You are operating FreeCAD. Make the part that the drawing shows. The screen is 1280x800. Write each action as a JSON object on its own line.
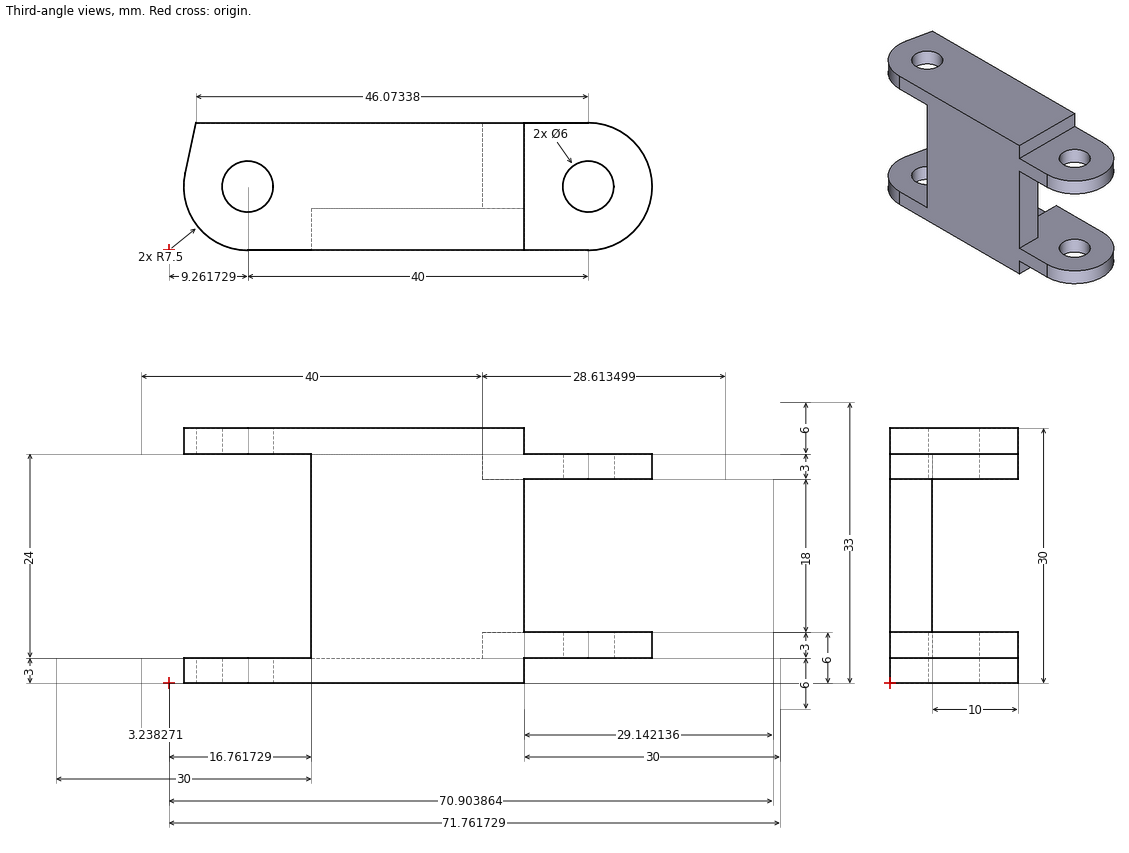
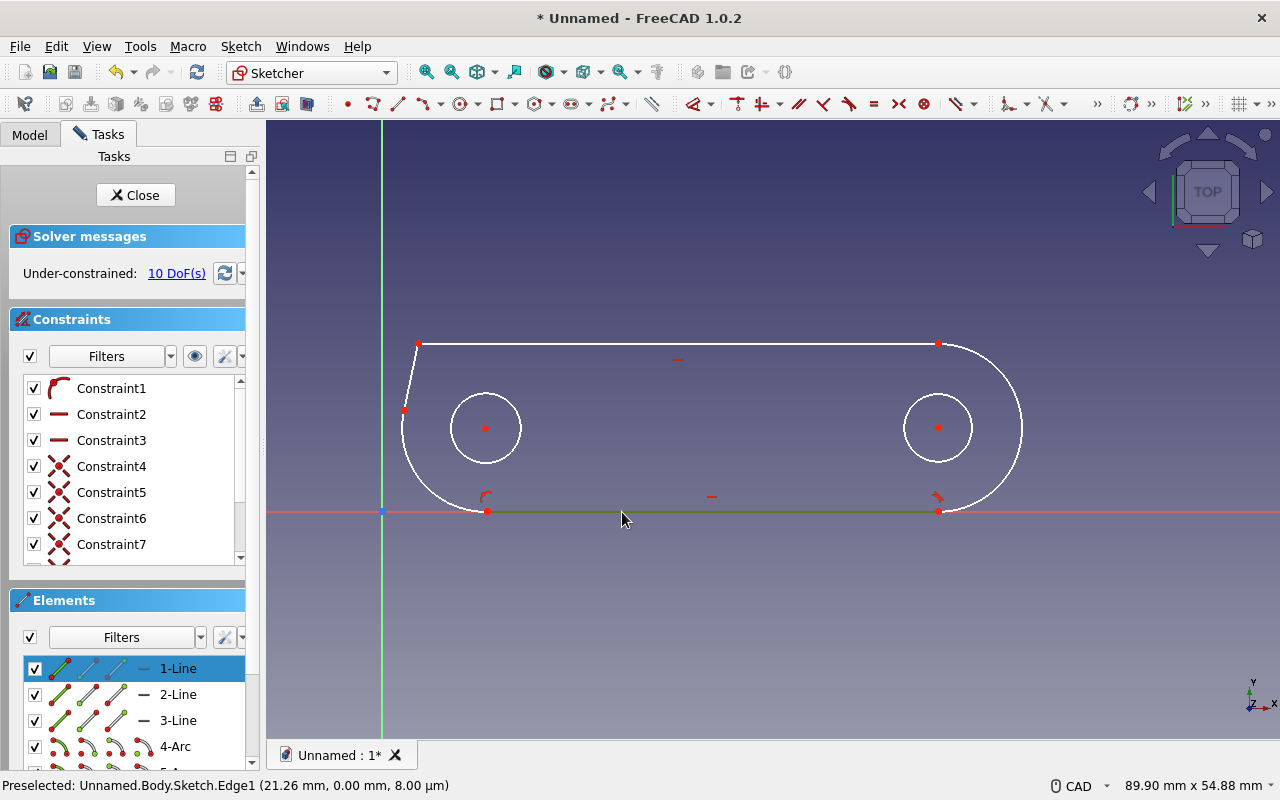
{"action": "left_click", "coordinate": [407, 455]}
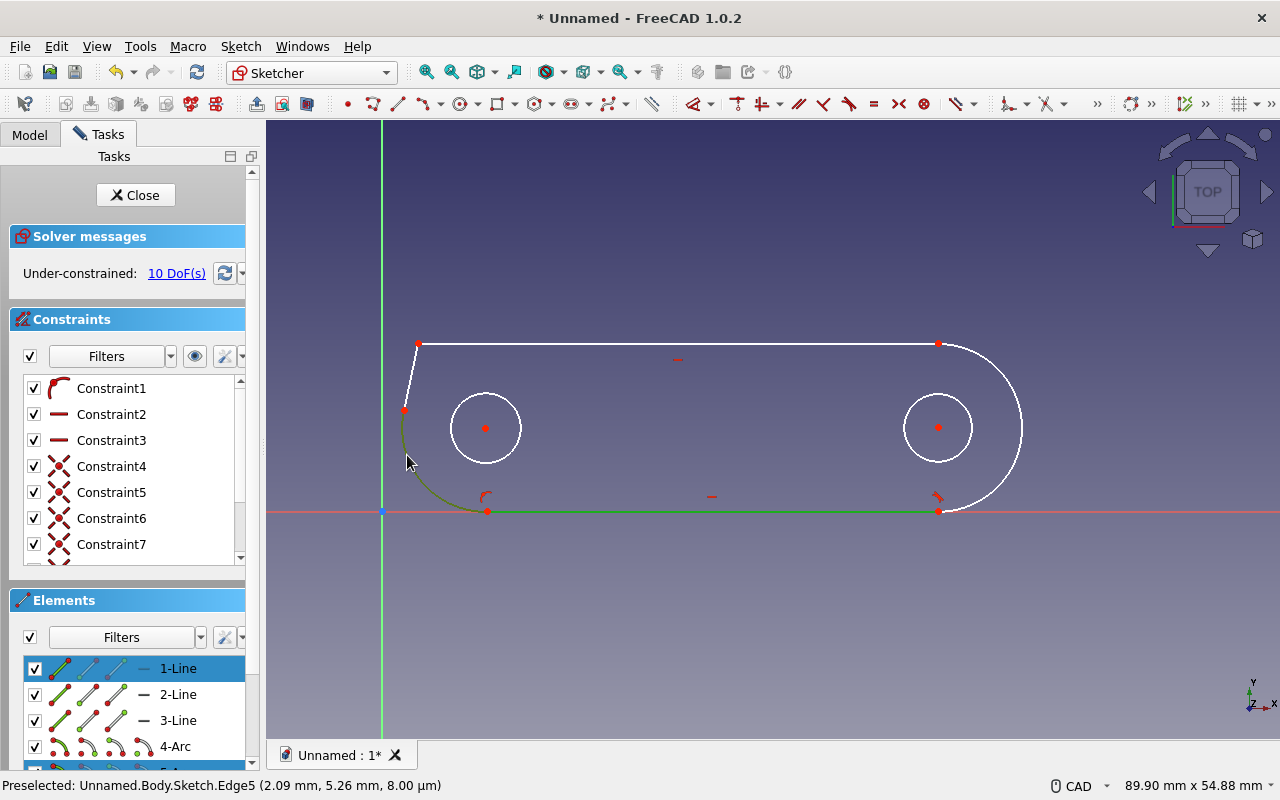
{"action": "left_click", "coordinate": [849, 104]}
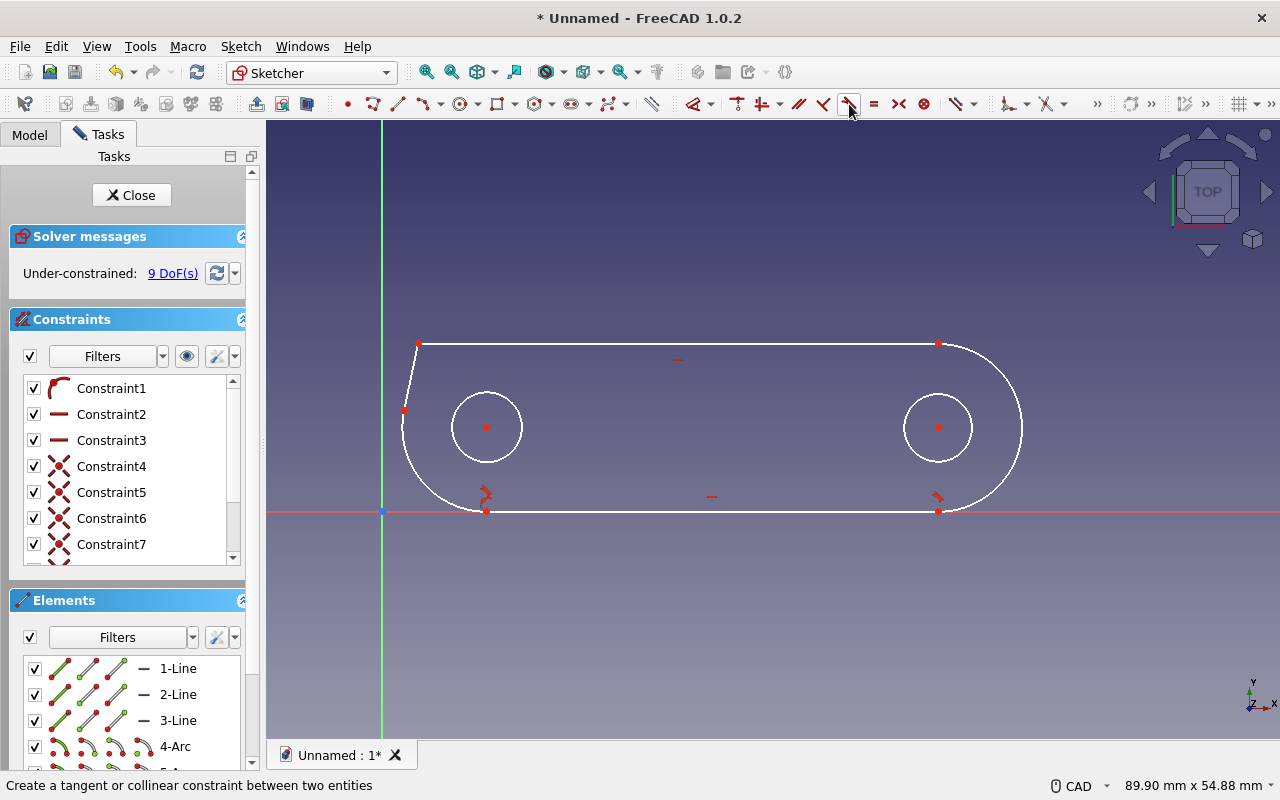
{"action": "left_click", "coordinate": [782, 344]}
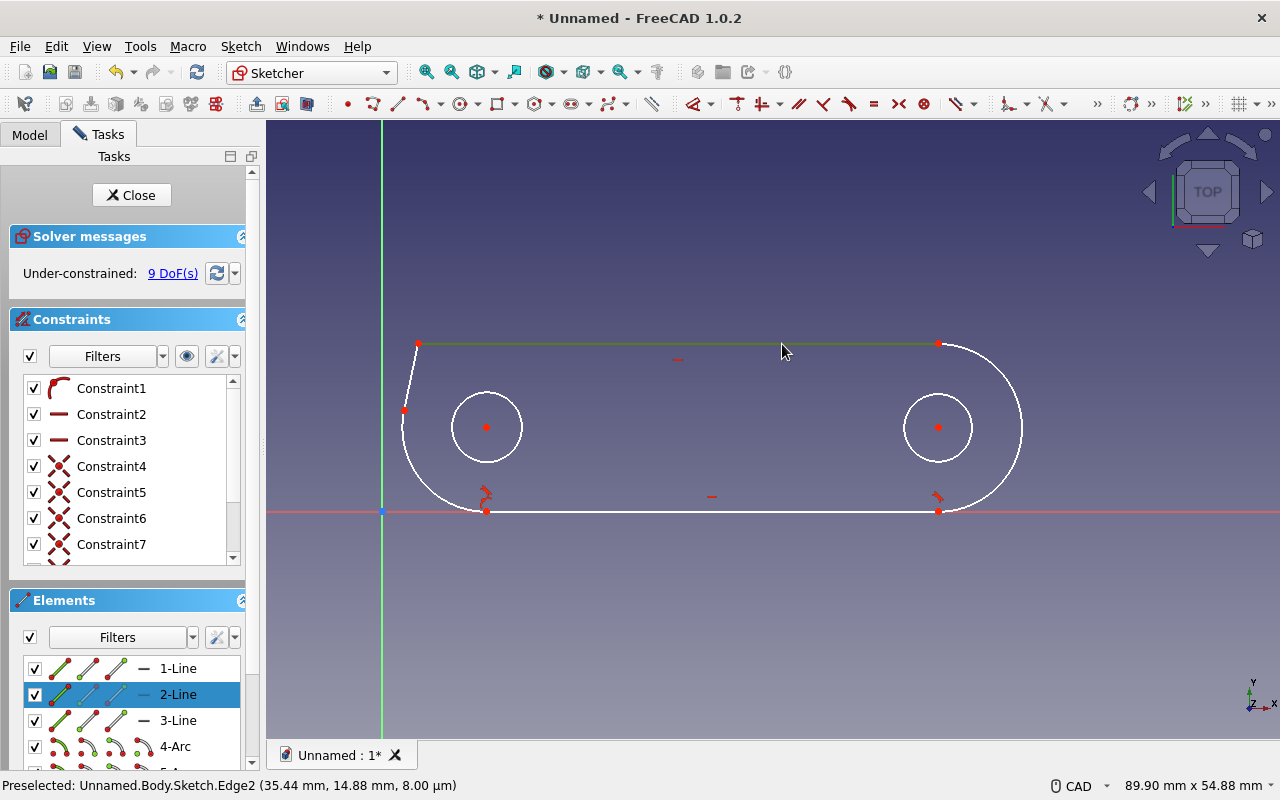
{"action": "left_click", "coordinate": [1006, 477]}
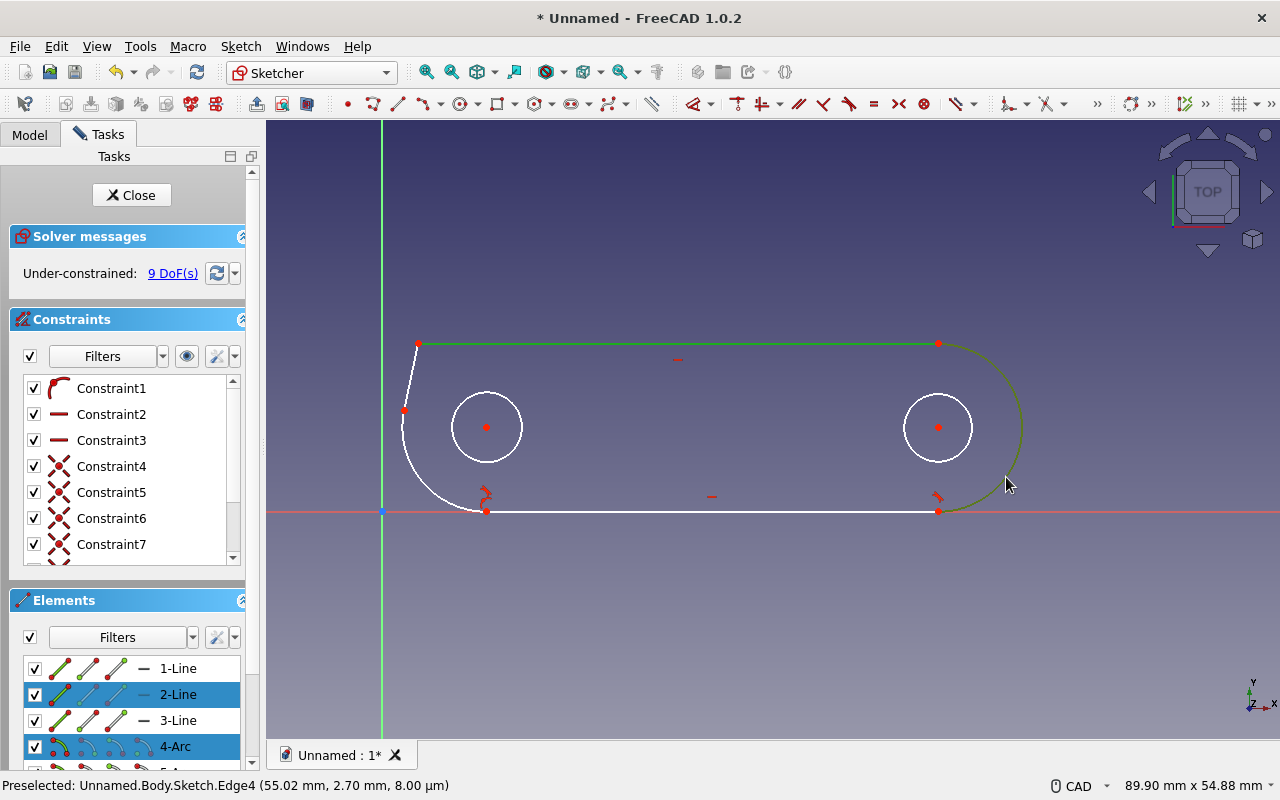
{"action": "key", "text": "t"}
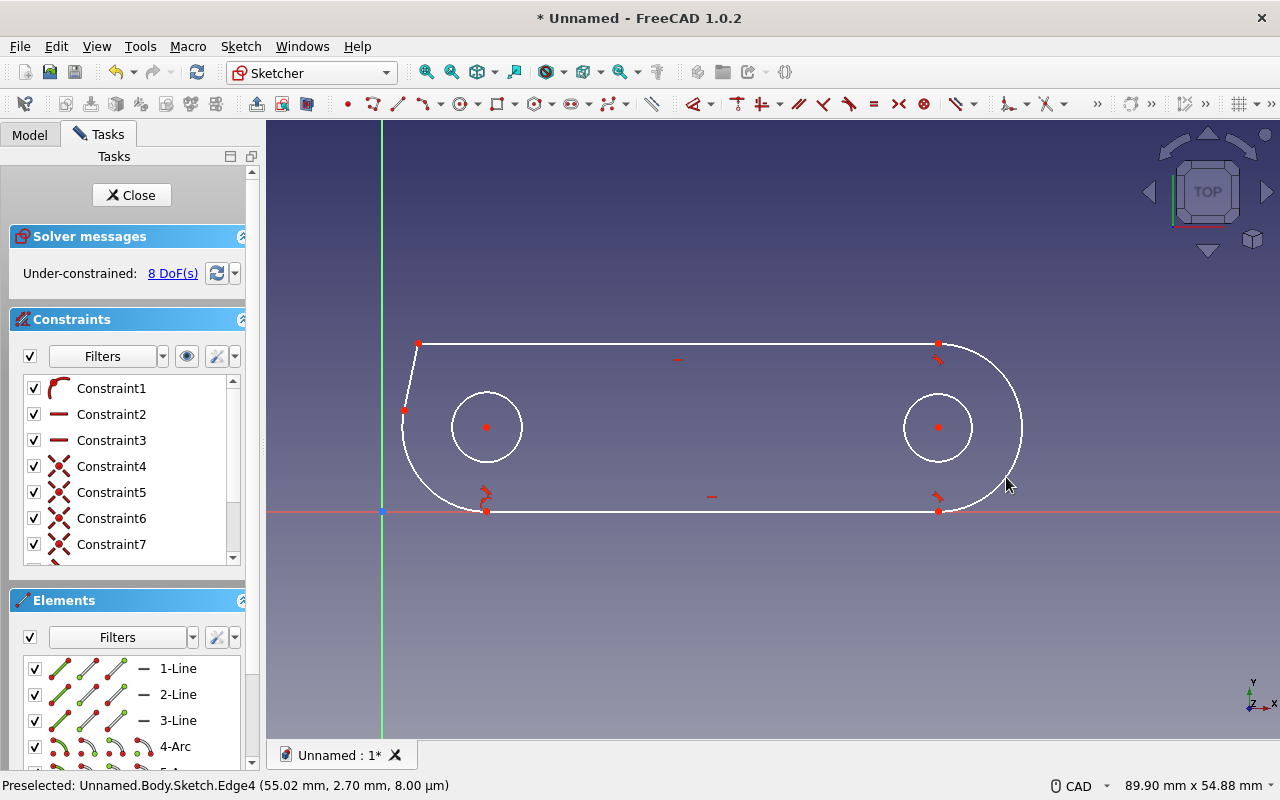
{"action": "left_click", "coordinate": [414, 364]}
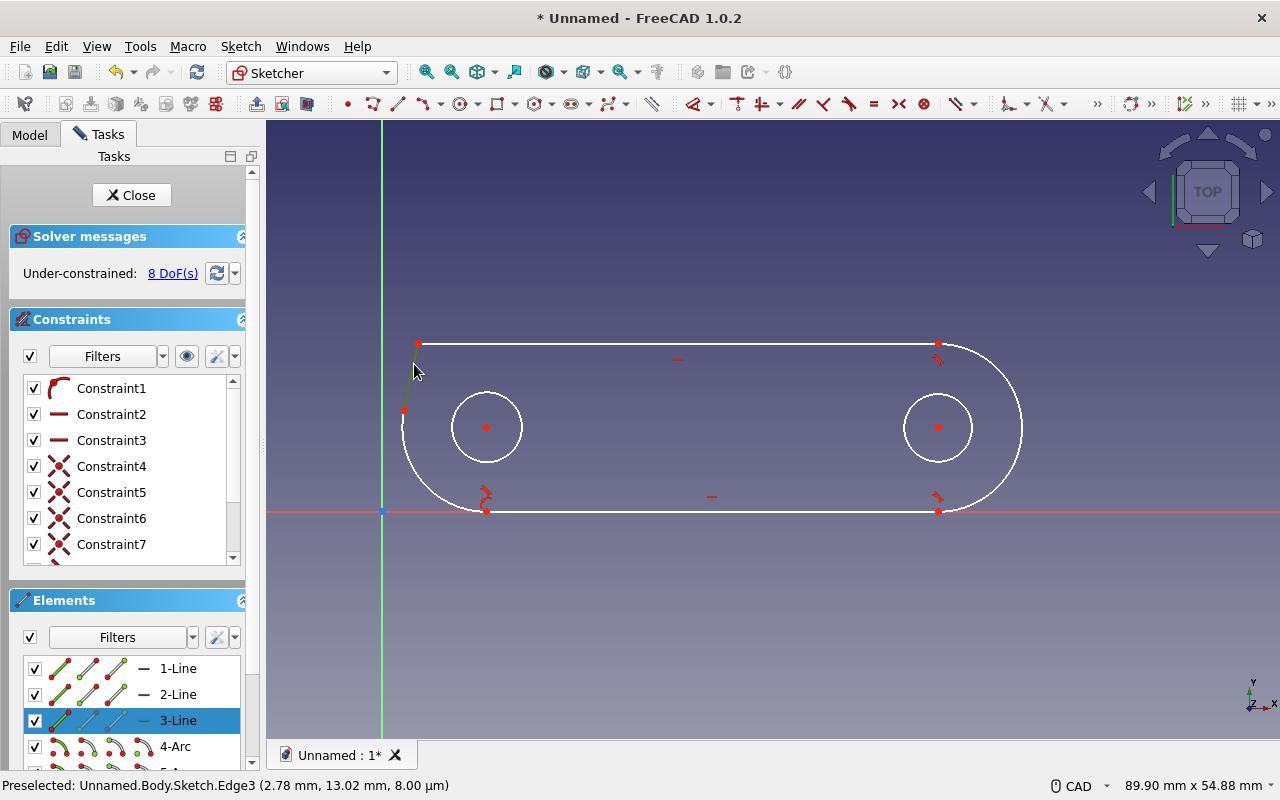
{"action": "left_click", "coordinate": [407, 455]}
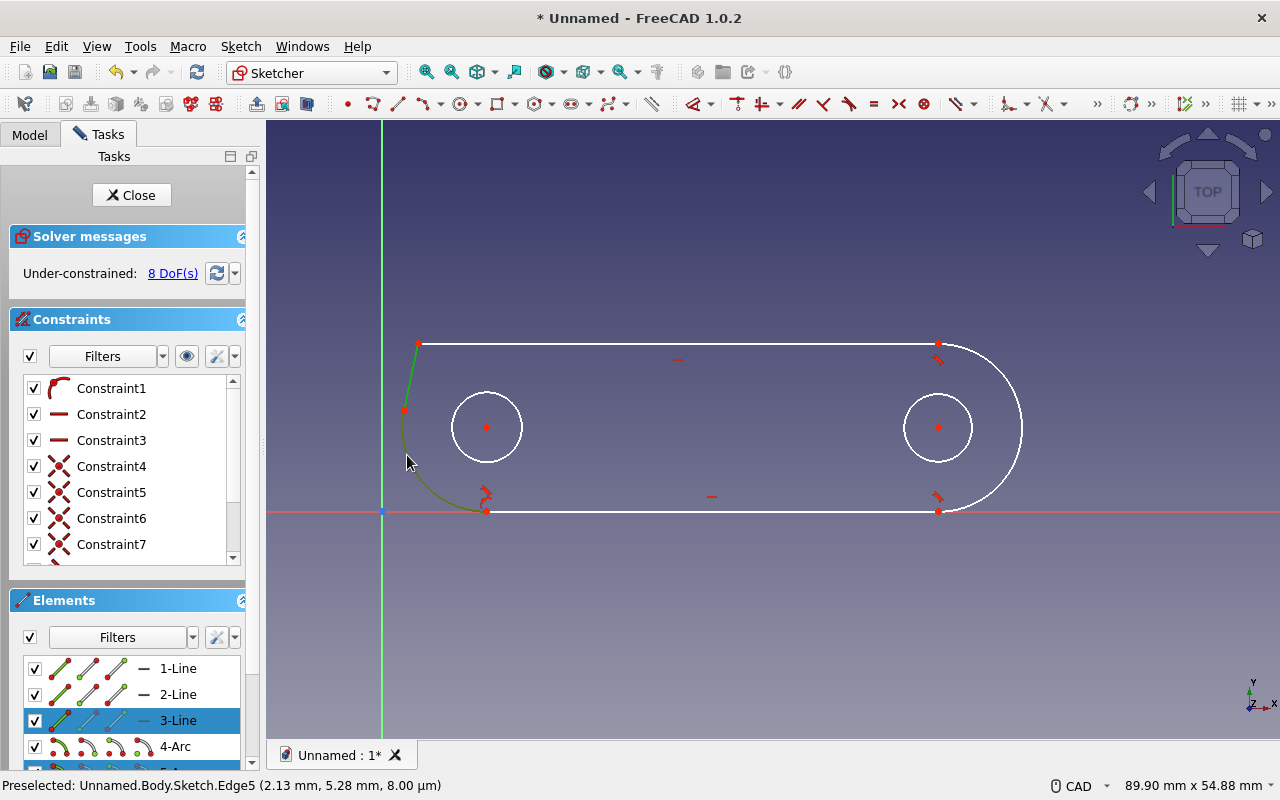
{"action": "left_click", "coordinate": [849, 104]}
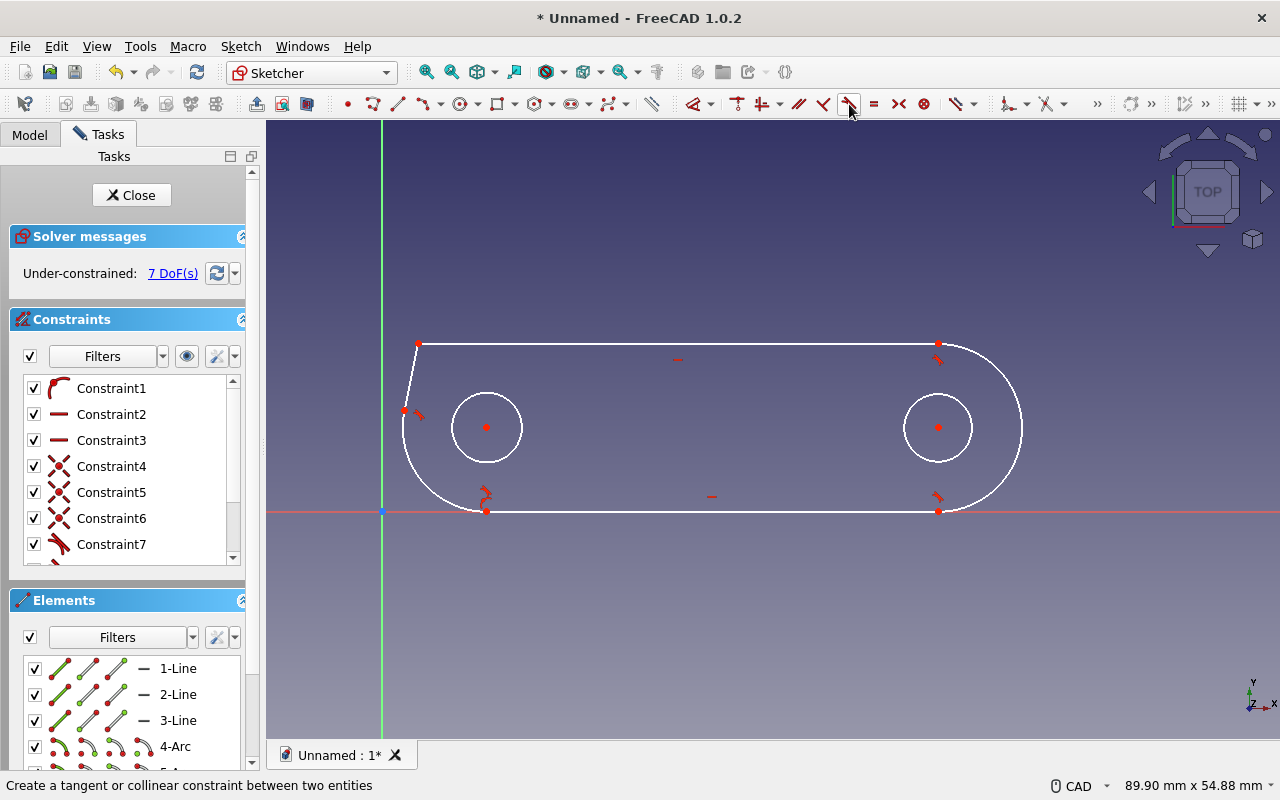
{"action": "left_click", "coordinate": [1006, 477]}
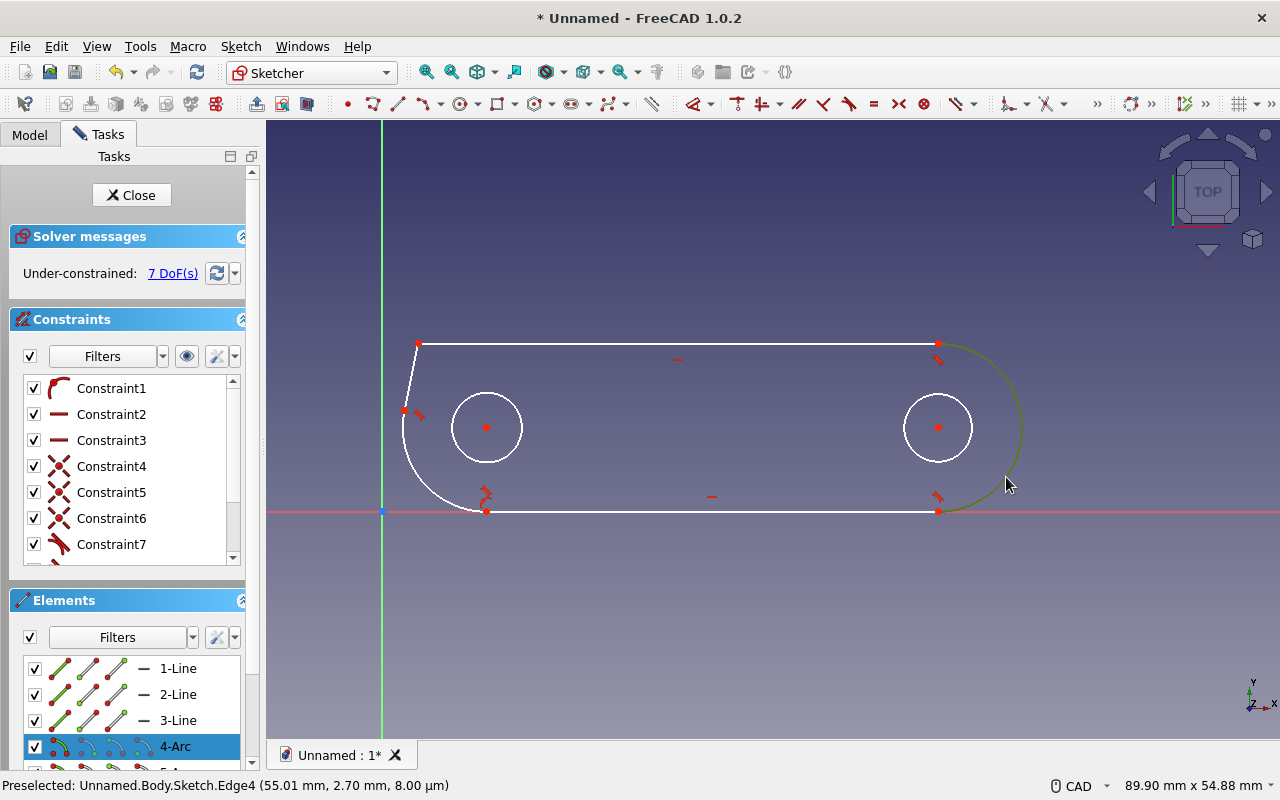
{"action": "left_click", "coordinate": [407, 455]}